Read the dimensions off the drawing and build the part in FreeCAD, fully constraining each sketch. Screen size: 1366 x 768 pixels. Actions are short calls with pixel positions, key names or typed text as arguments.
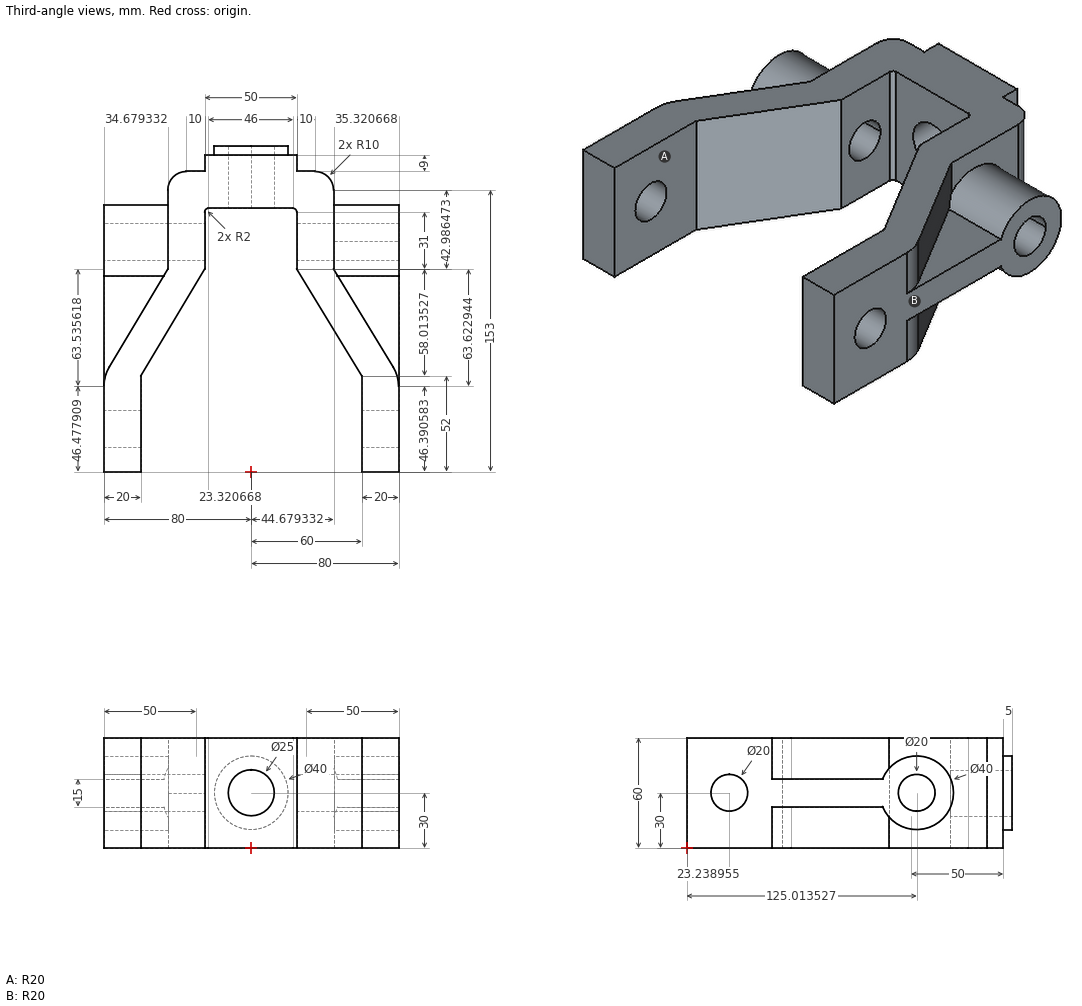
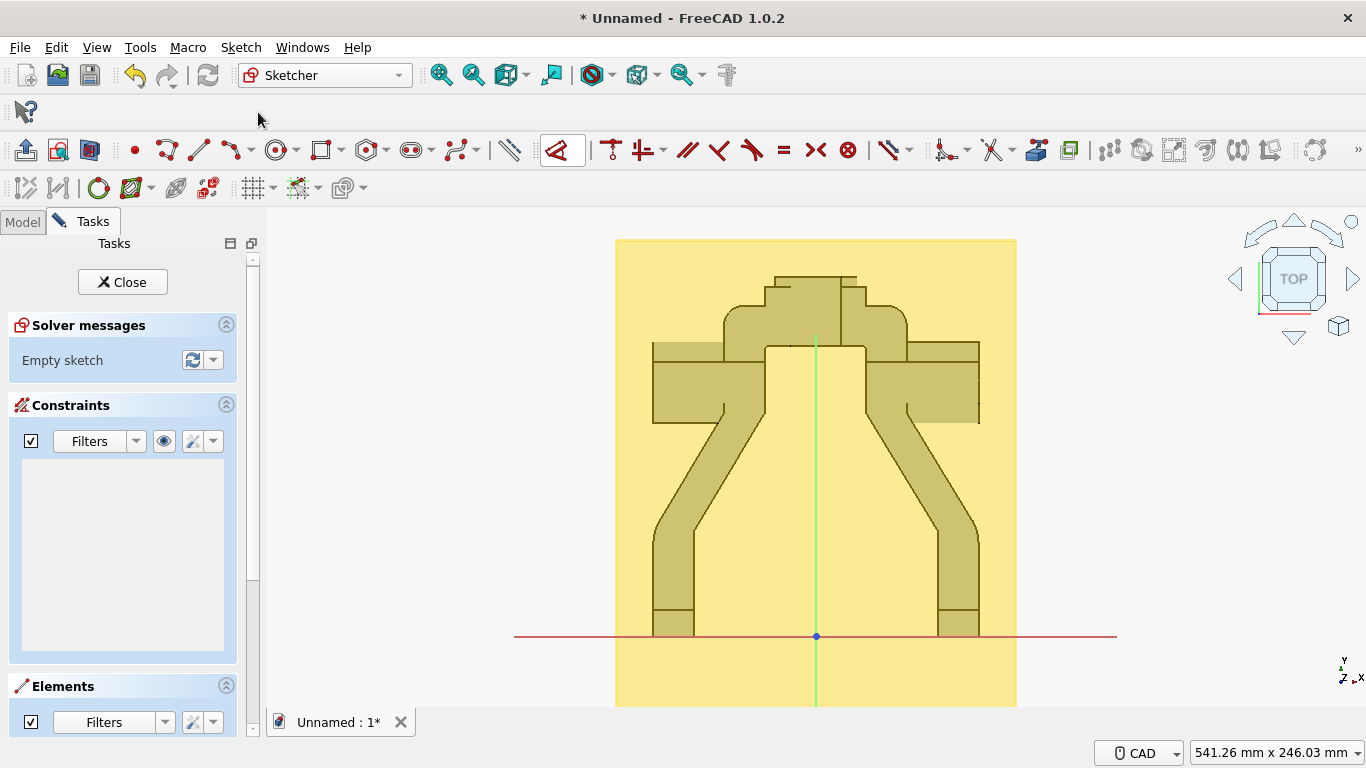
scroll(955, 663, up, 2)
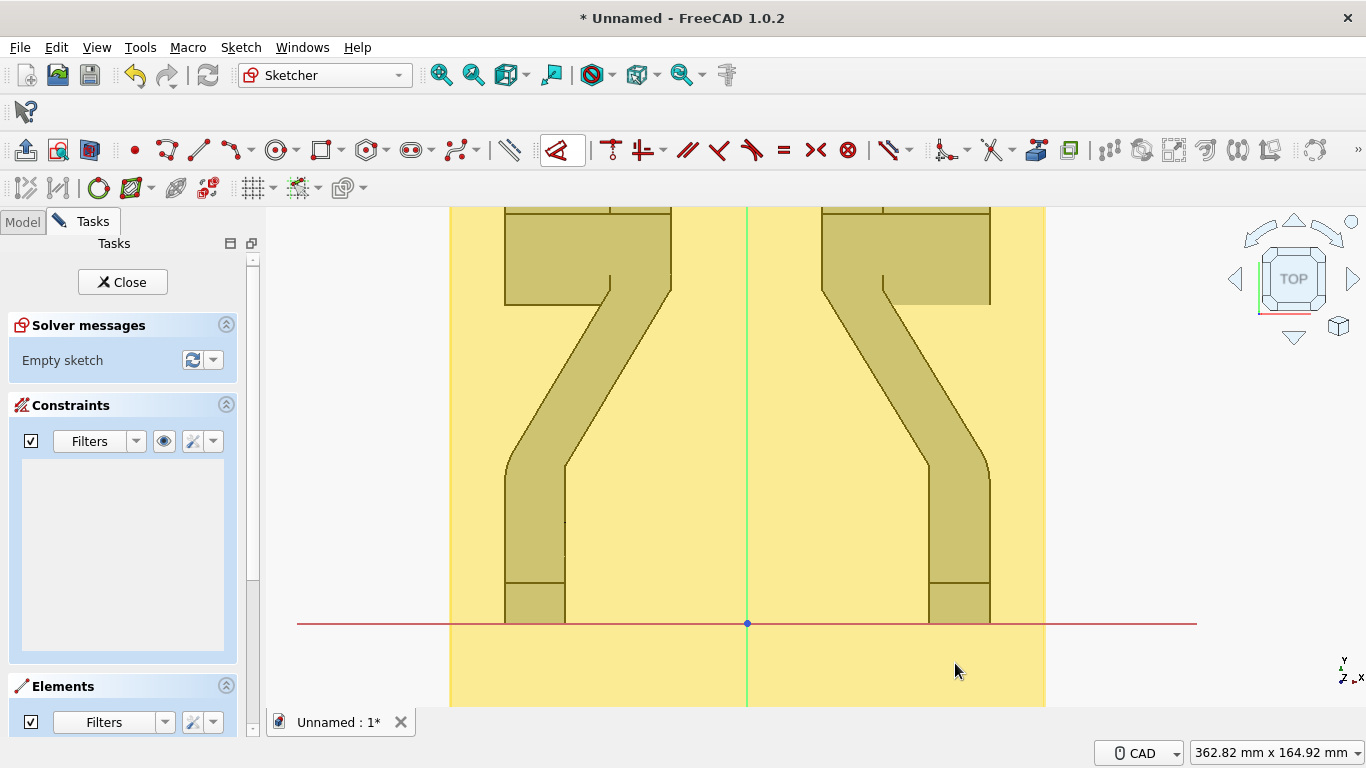
key(g)
key(m)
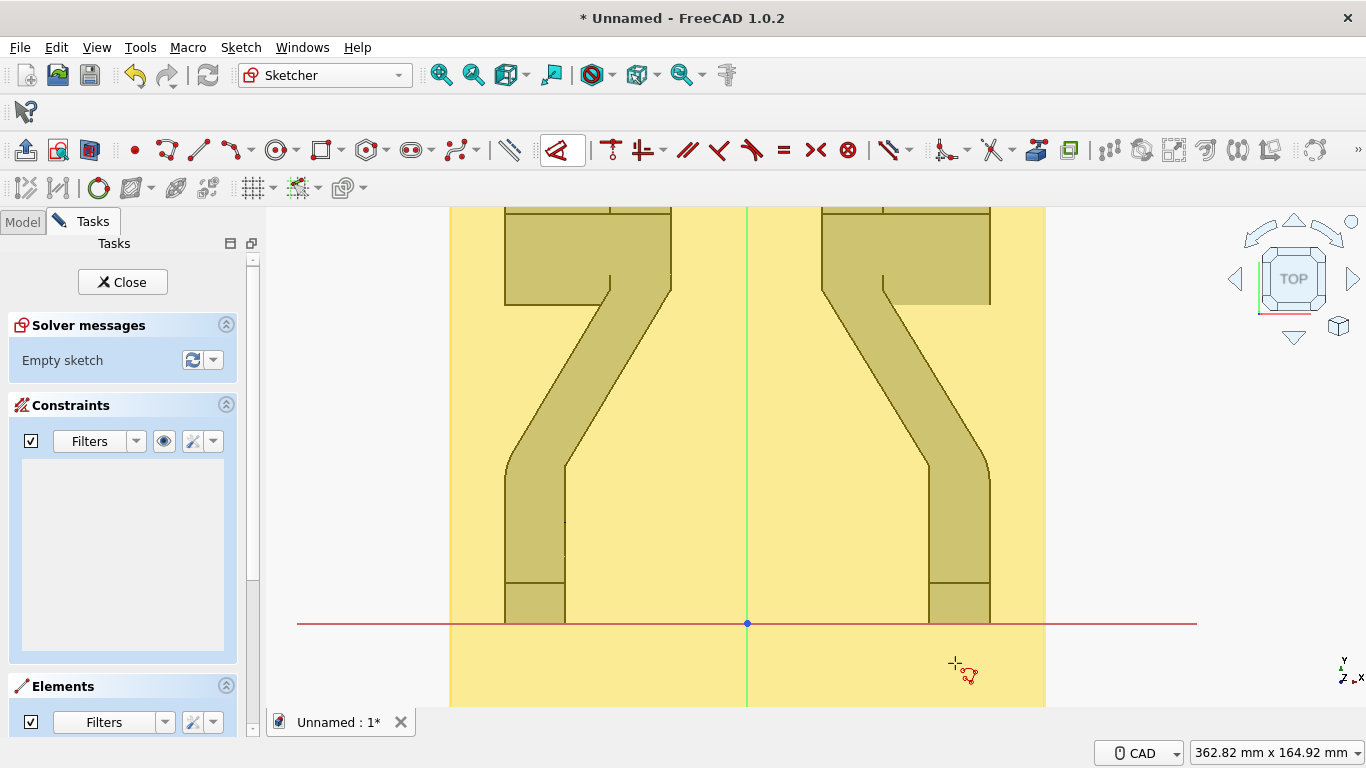
click(505, 483)
click(610, 290)
click(505, 290)
click(505, 484)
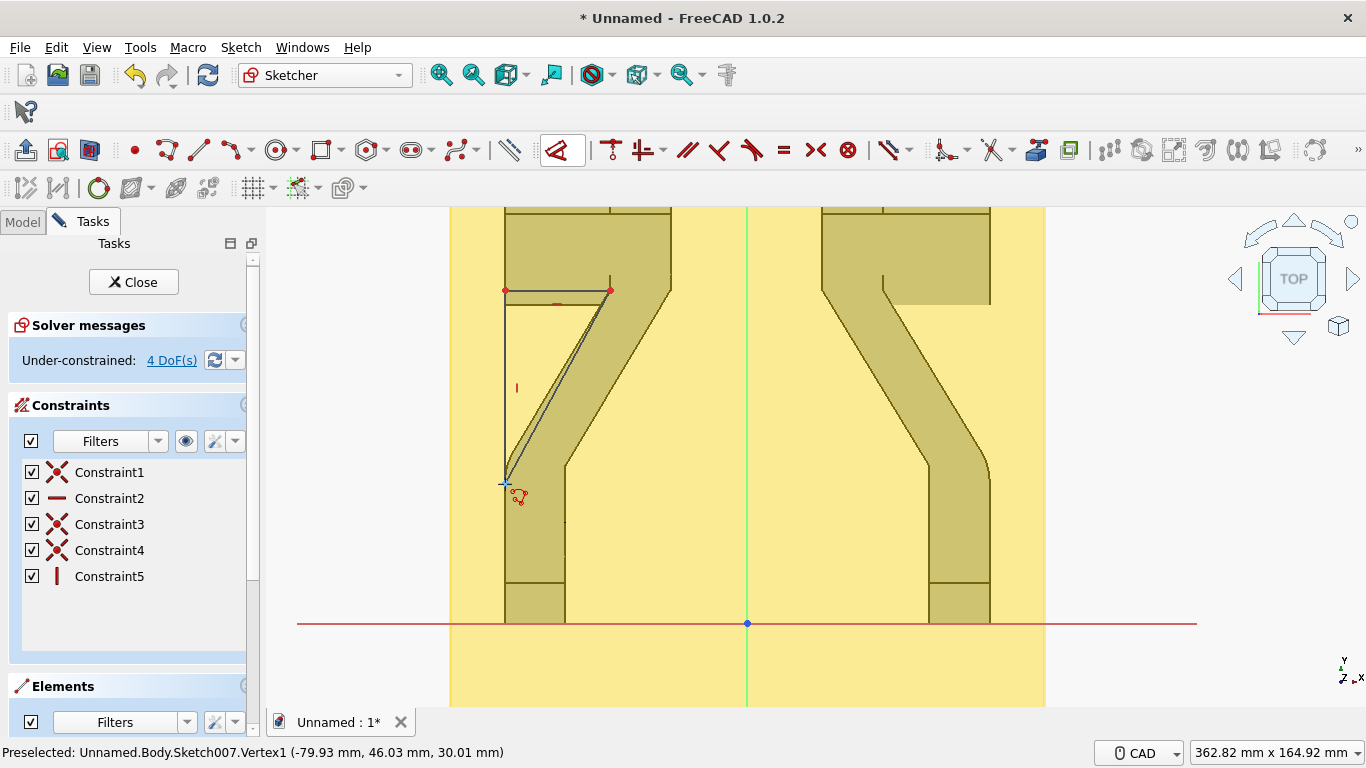
click(990, 483)
click(990, 290)
click(883, 290)
click(990, 484)
key(Escape)
key(Escape)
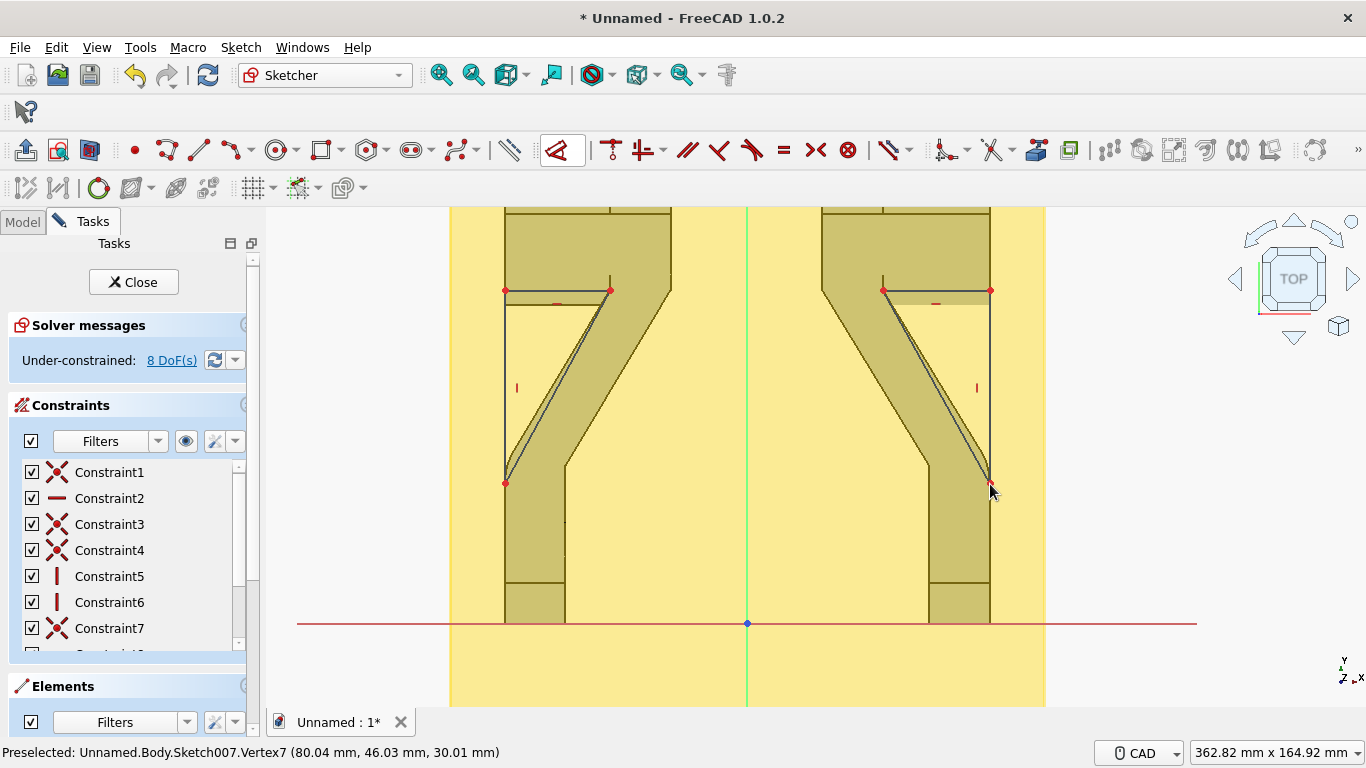
click(505, 484)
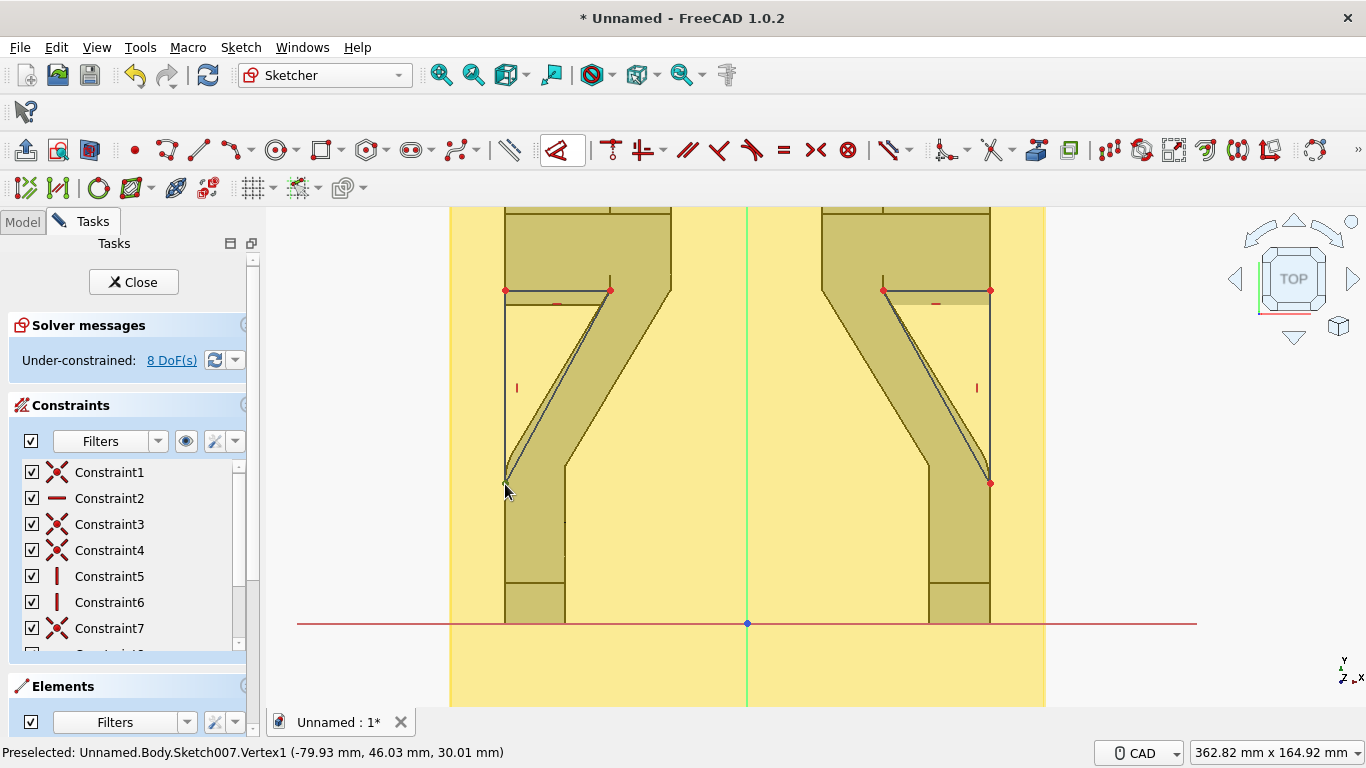
key(l)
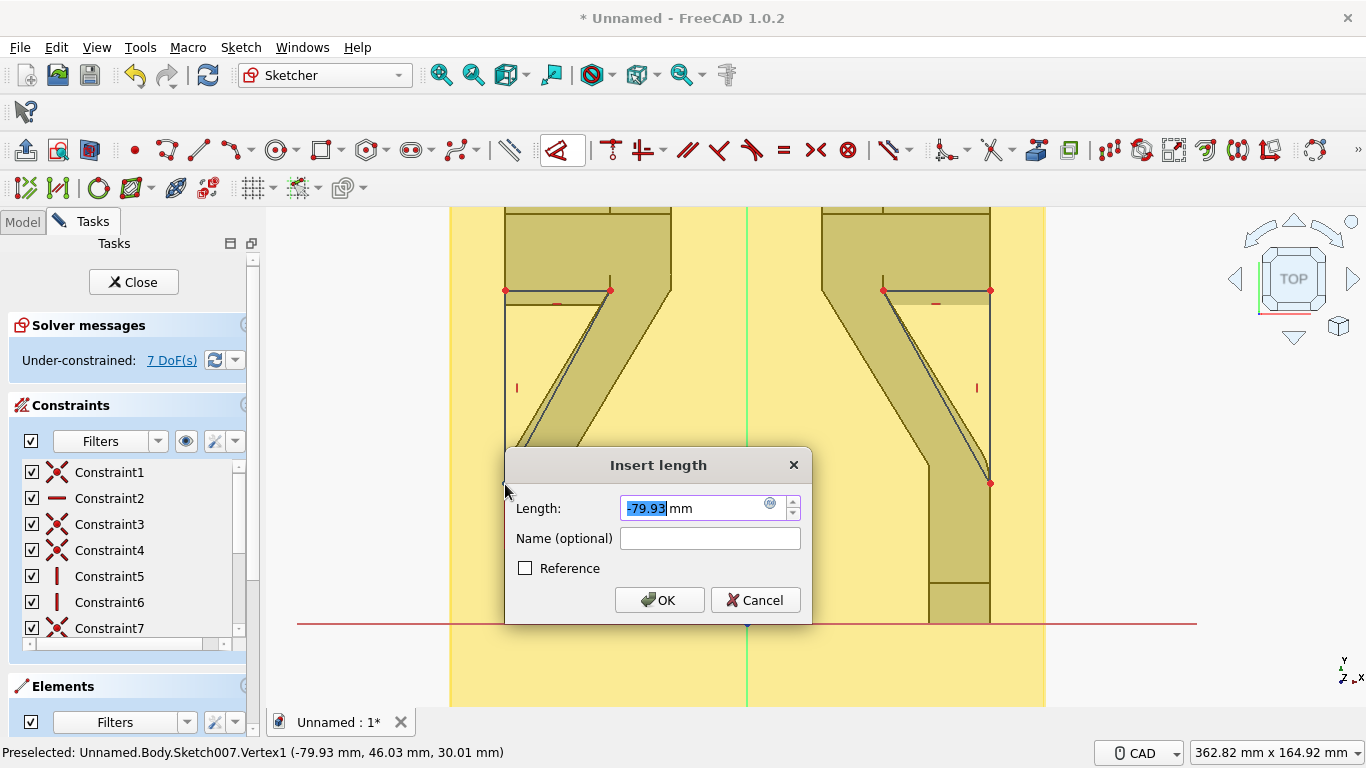
text(-80)
key(Return)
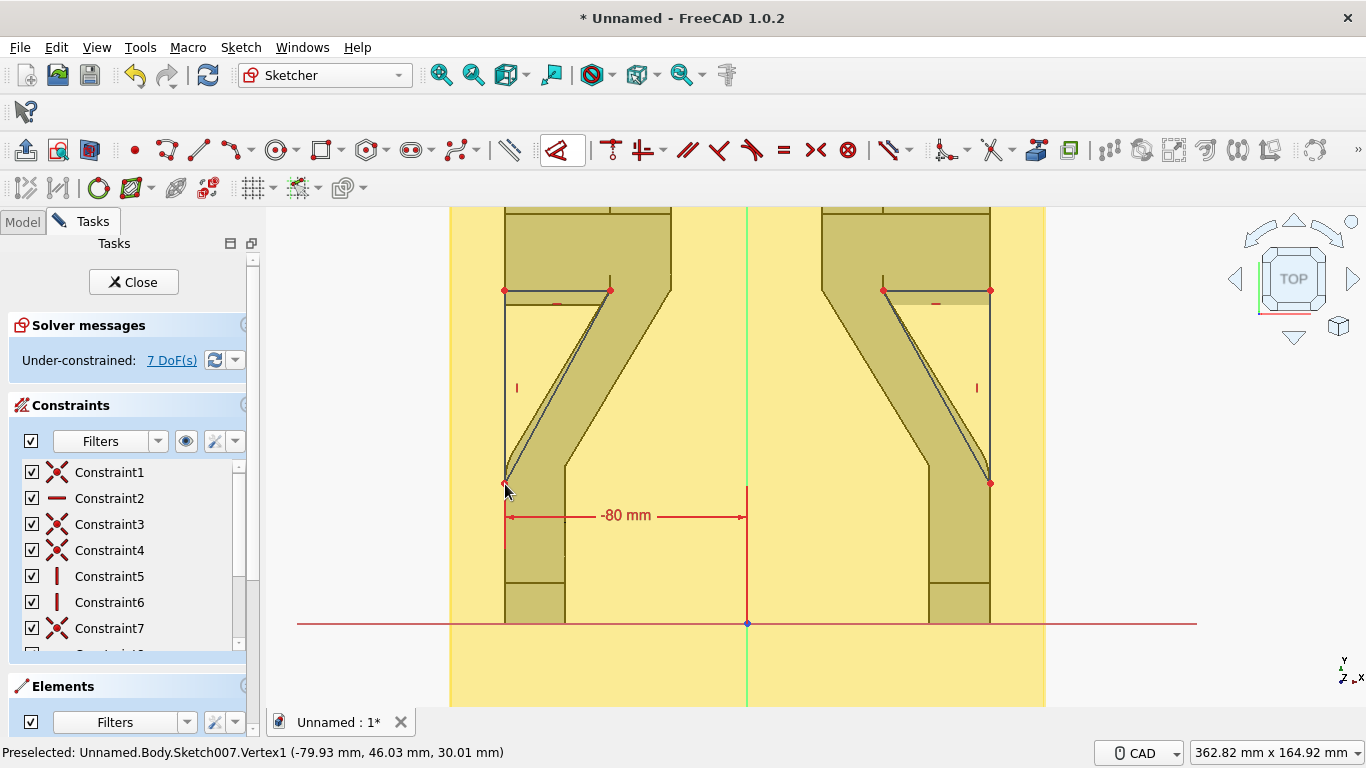
click(990, 484)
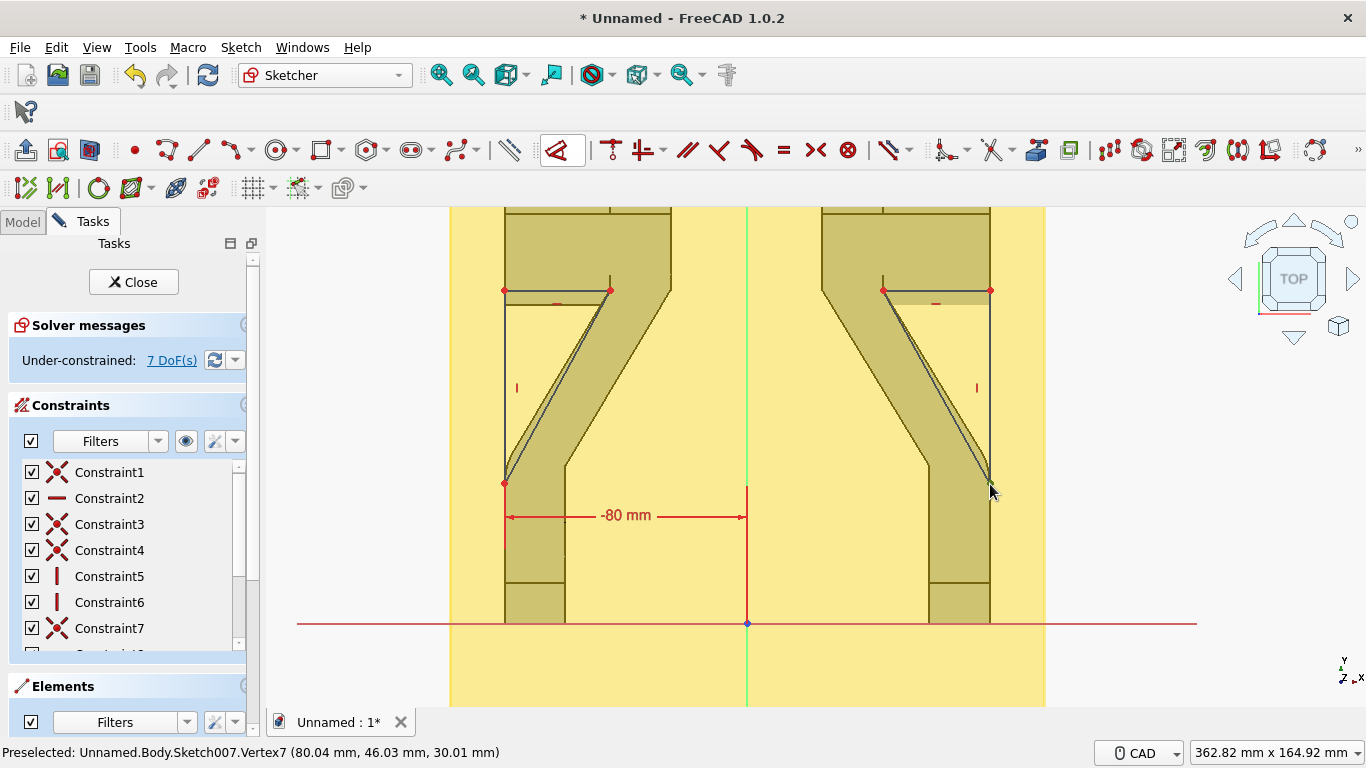
key(l)